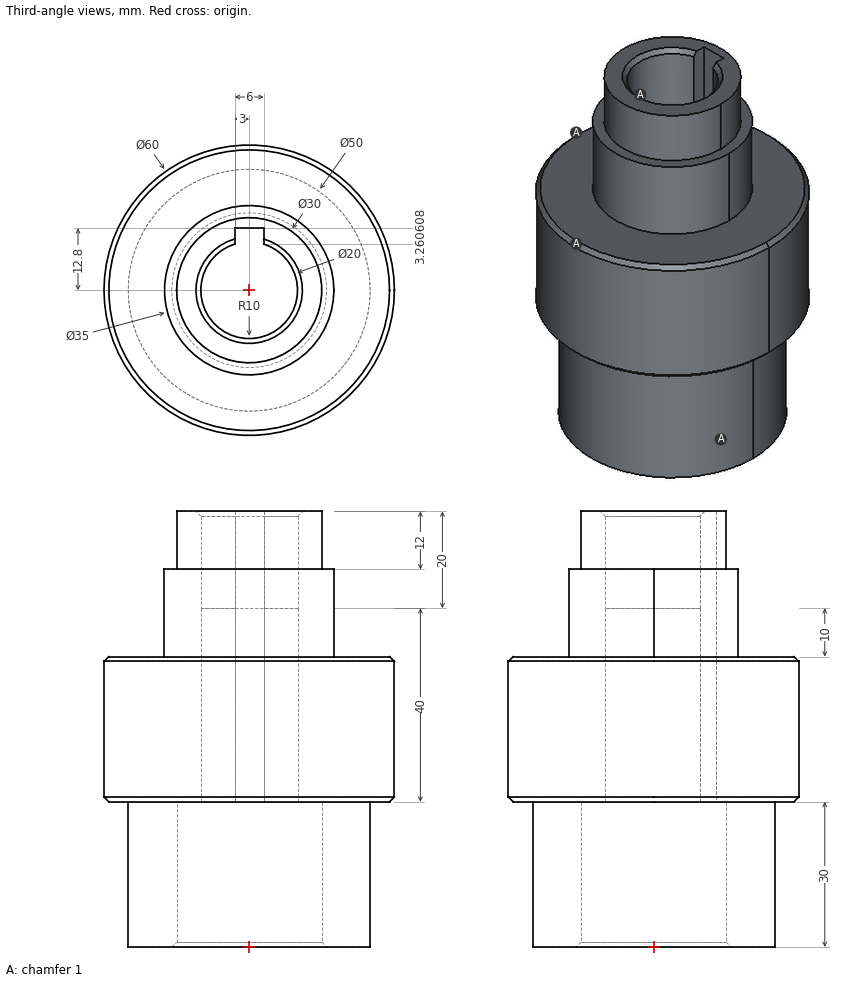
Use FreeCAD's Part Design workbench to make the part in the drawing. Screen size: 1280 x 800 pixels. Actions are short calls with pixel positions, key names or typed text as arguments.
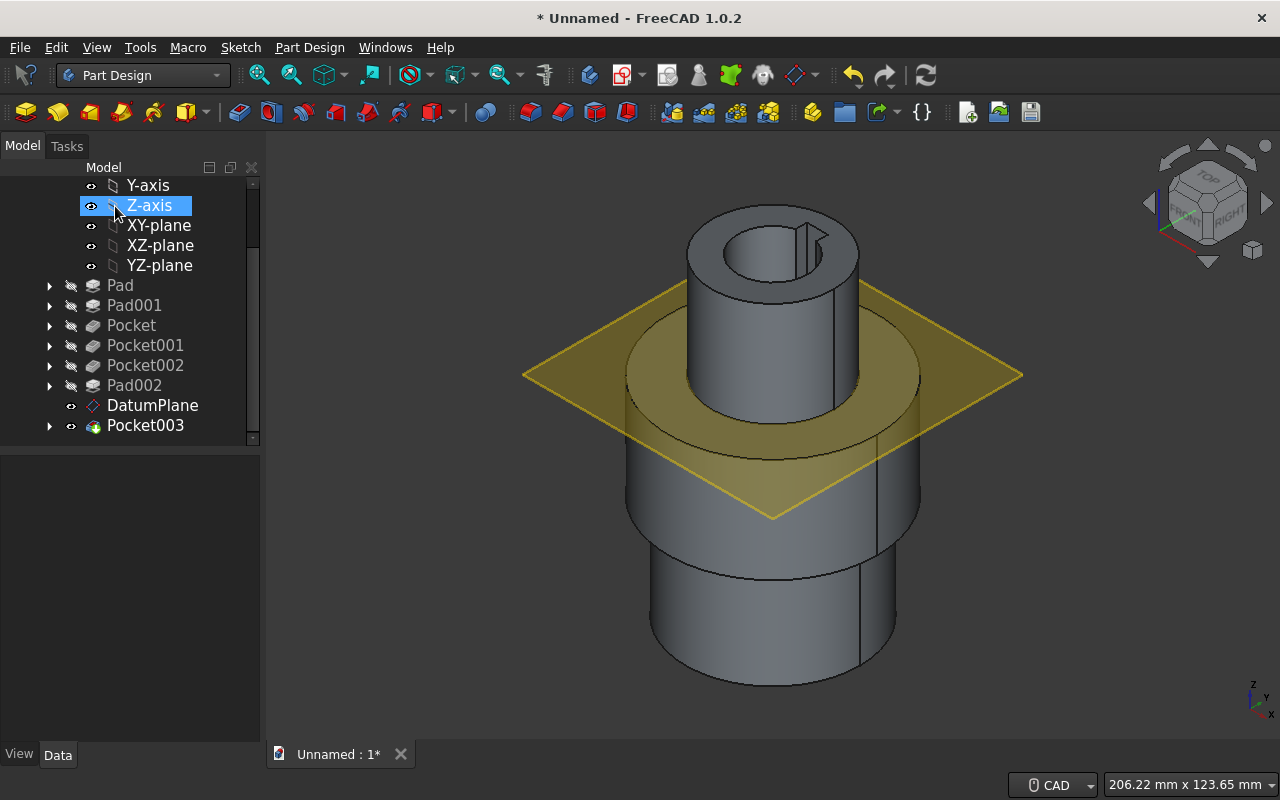
click(116, 406)
key(space)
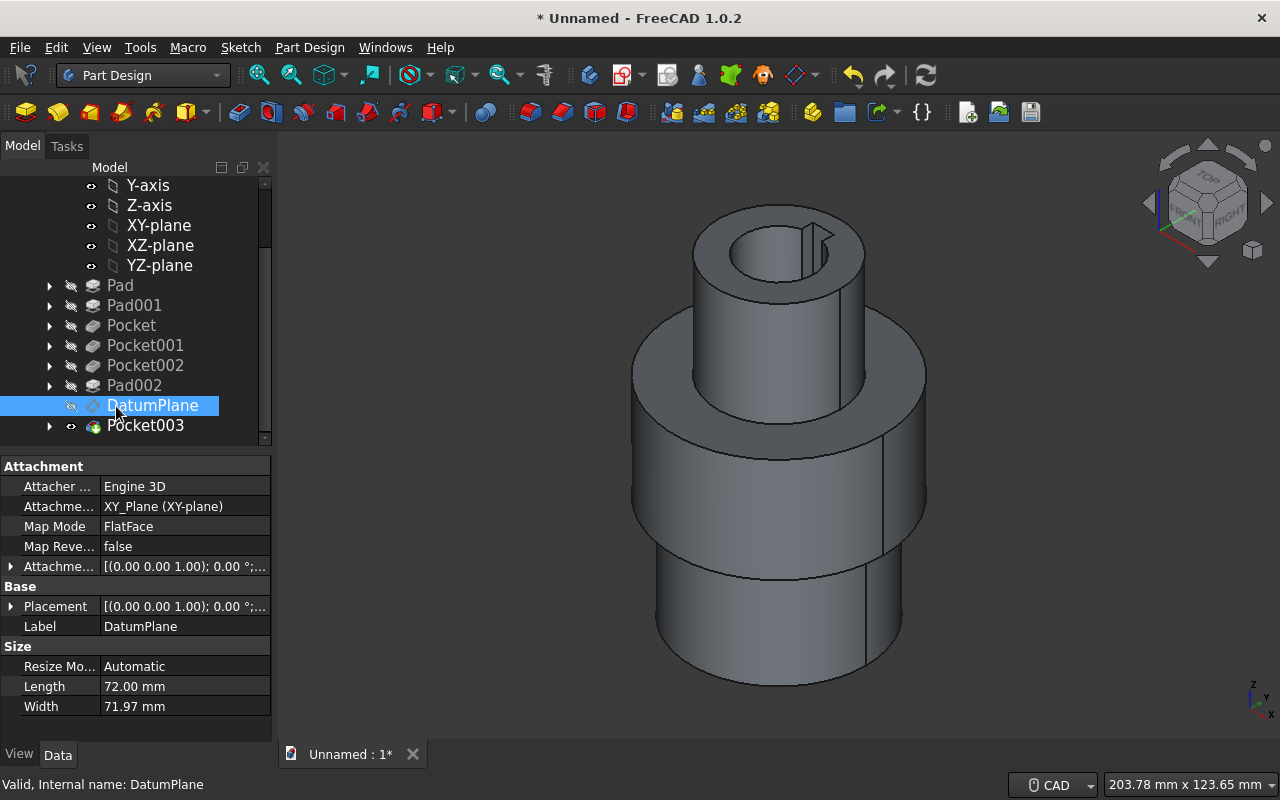
scroll(160, 301, down, 3)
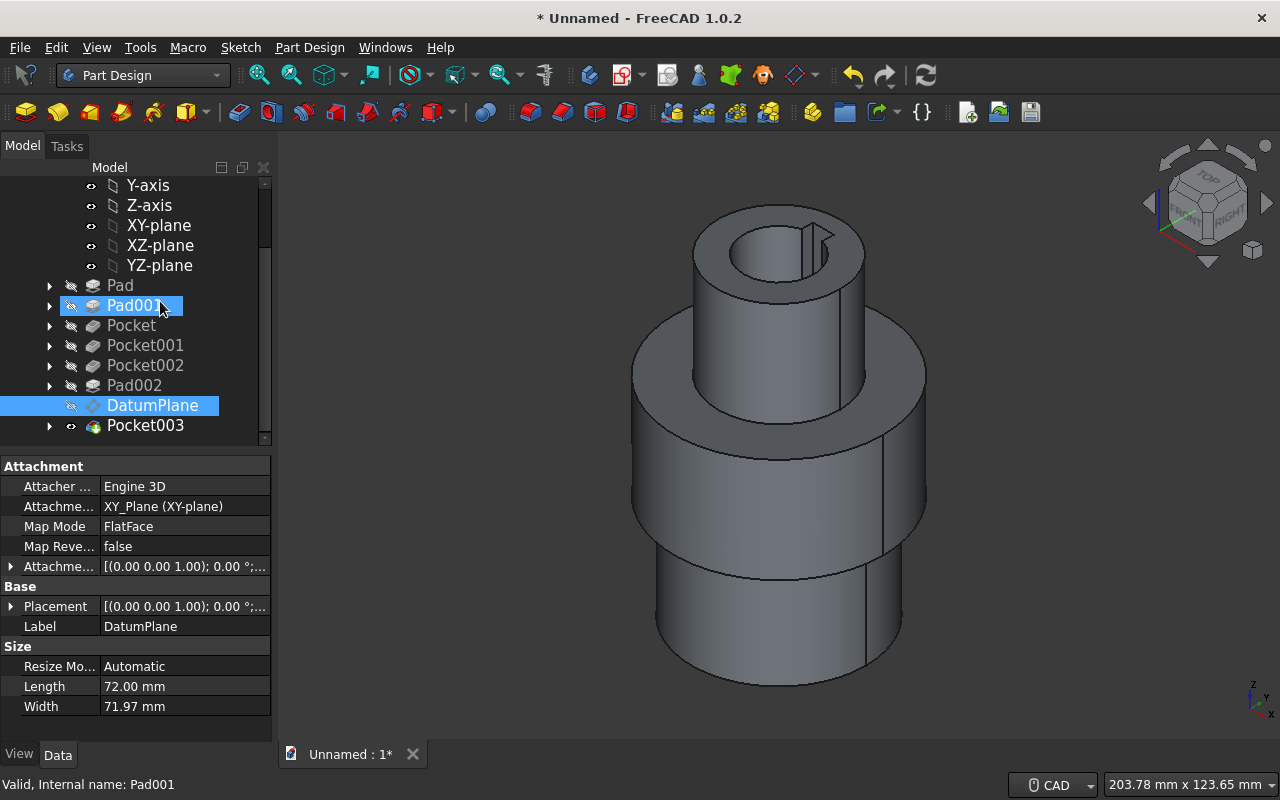
scroll(160, 301, up, 15)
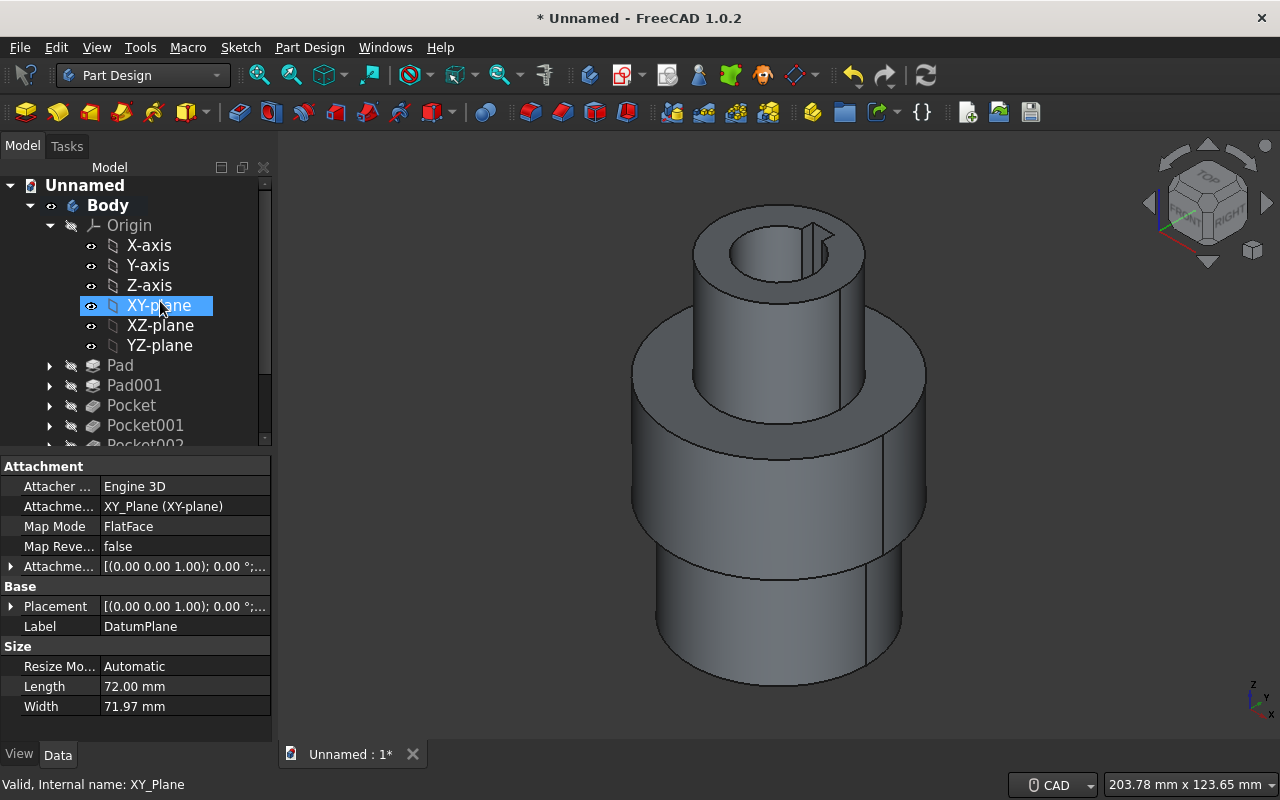
click(136, 306)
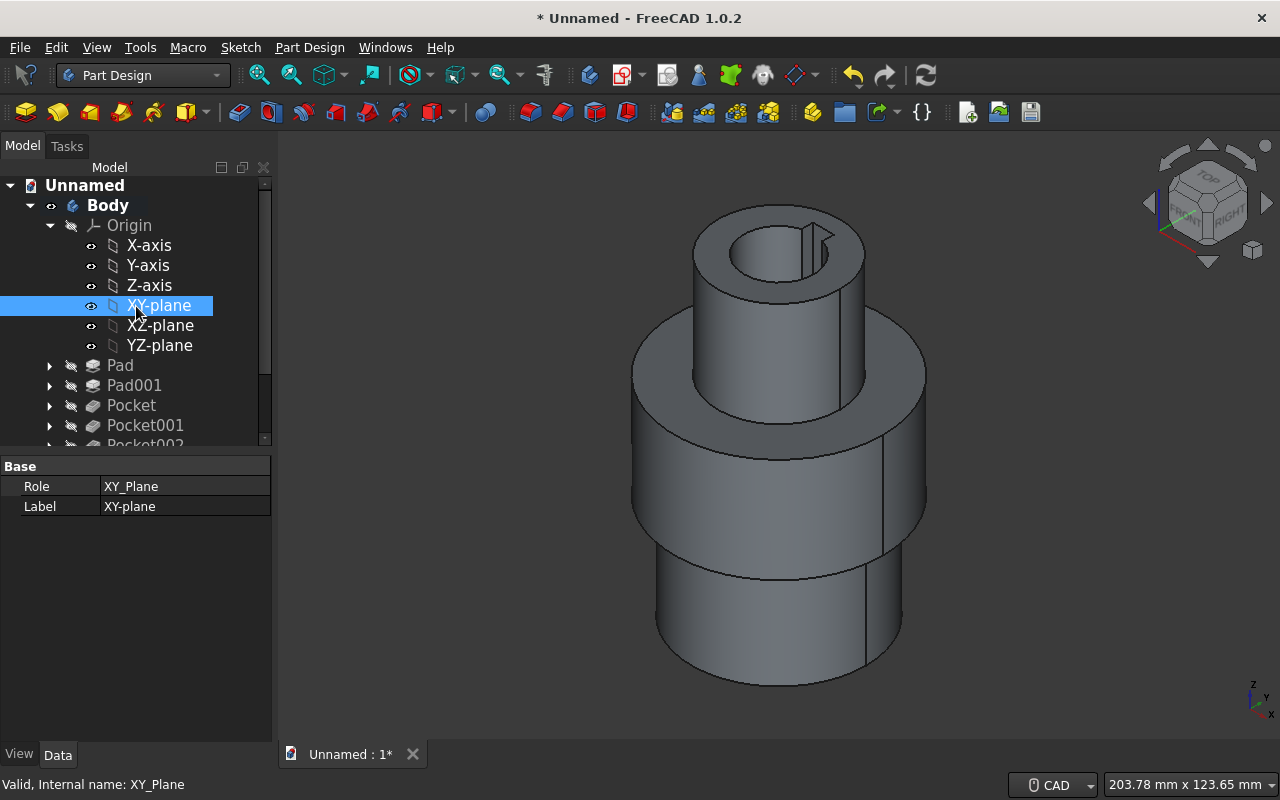
click(796, 76)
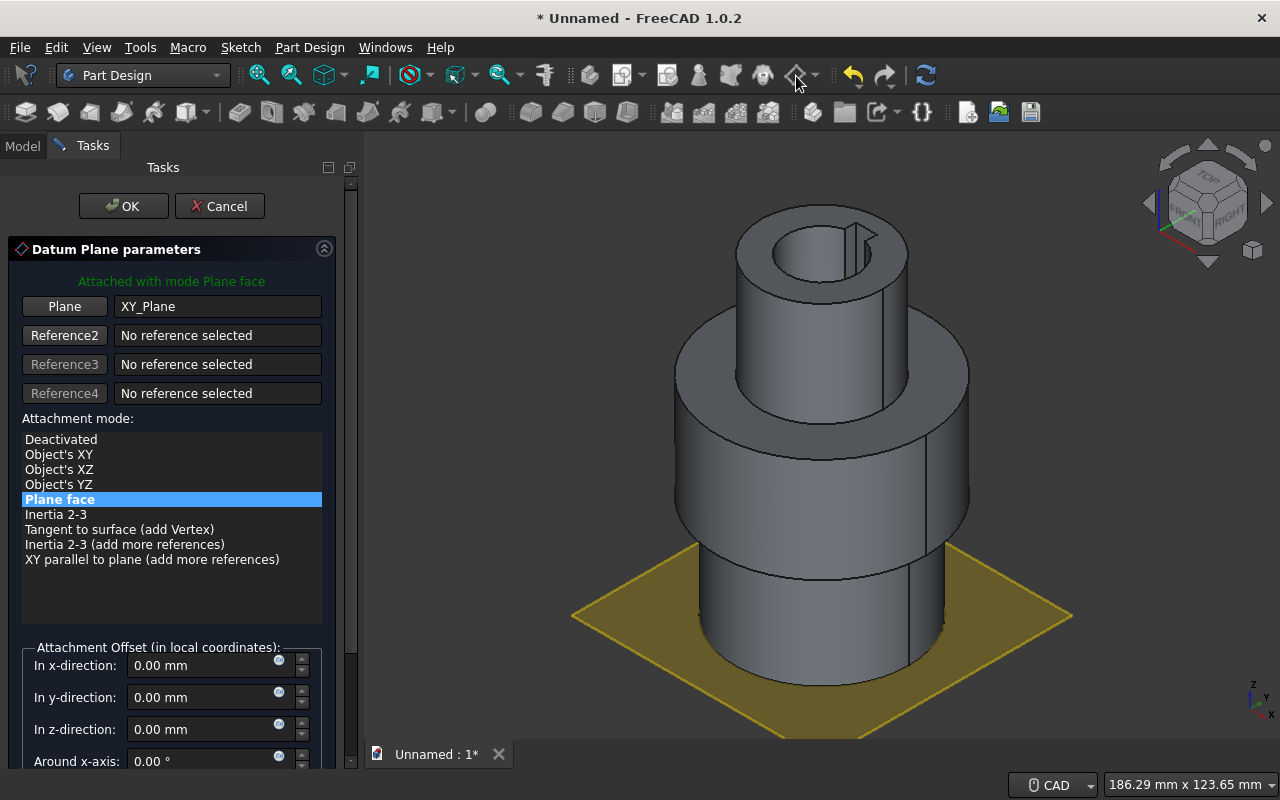
triple_click(210, 729)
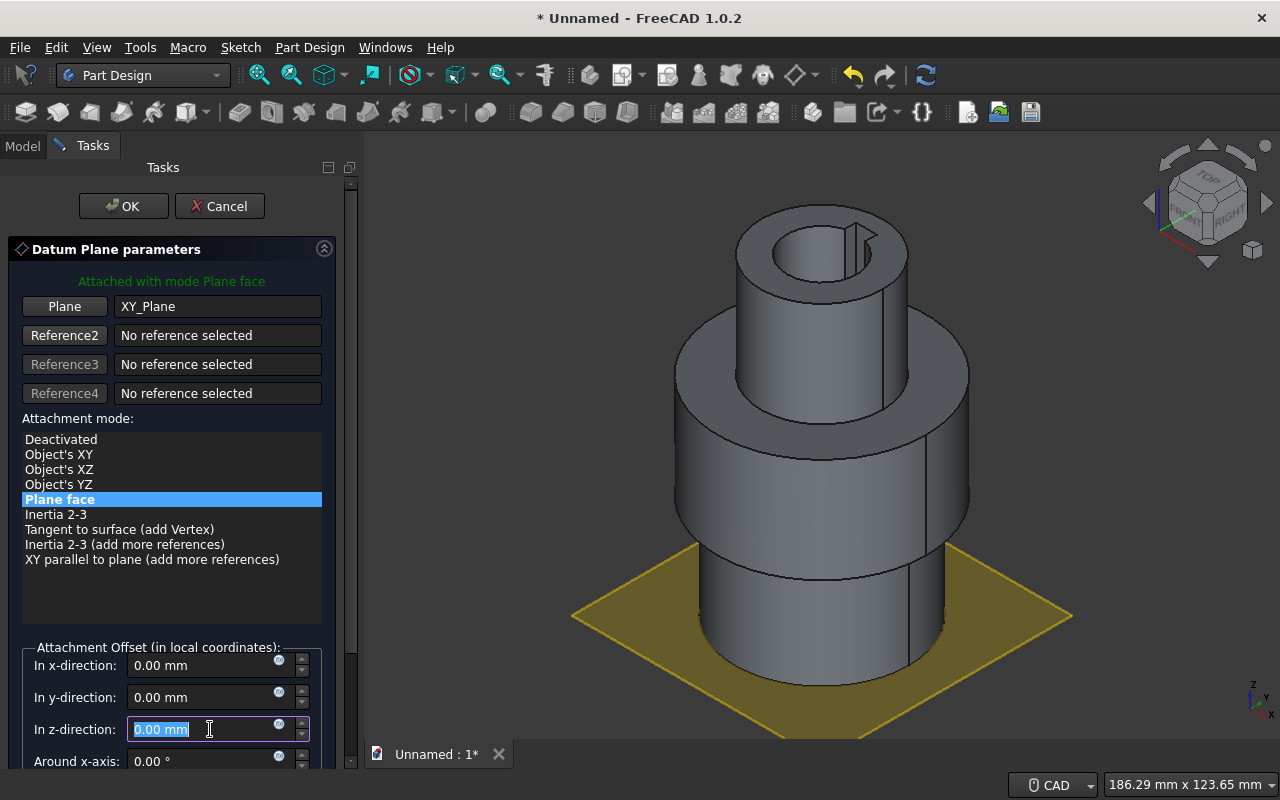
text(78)
key(Tab)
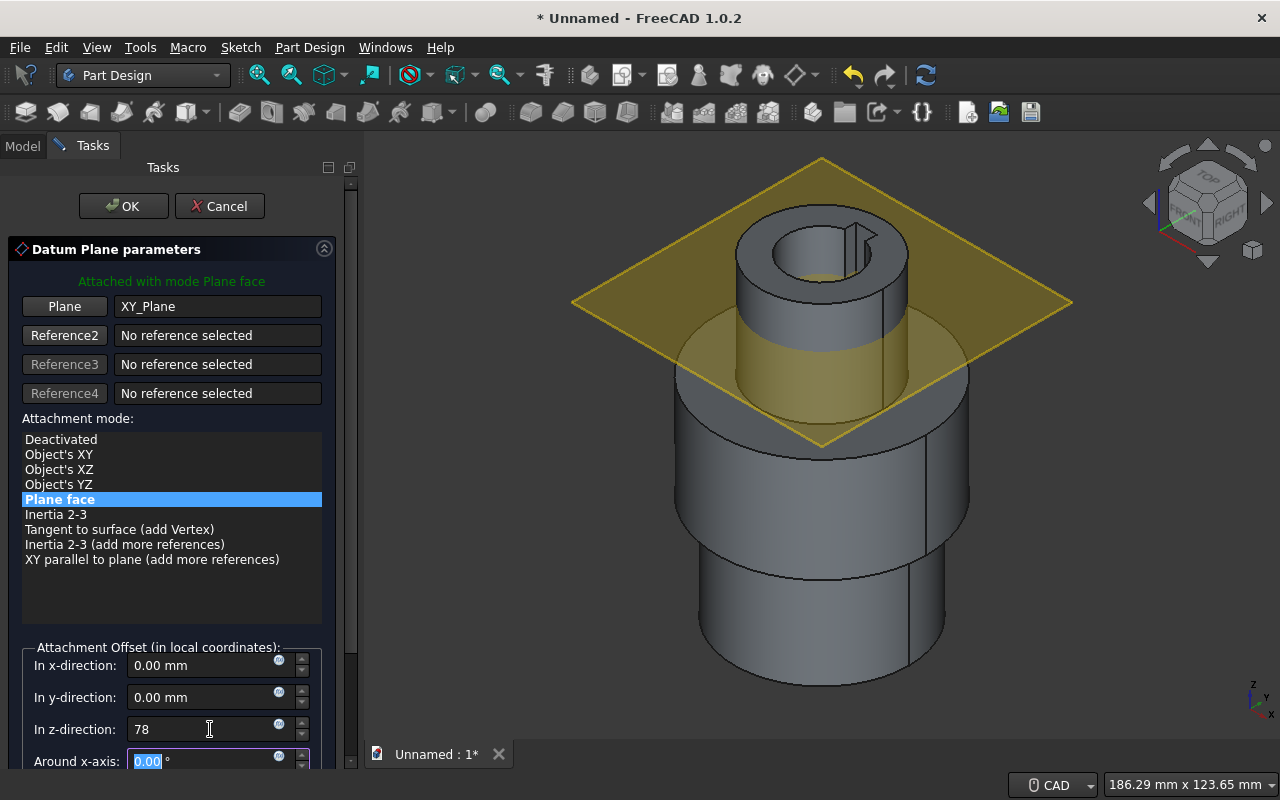
click(124, 206)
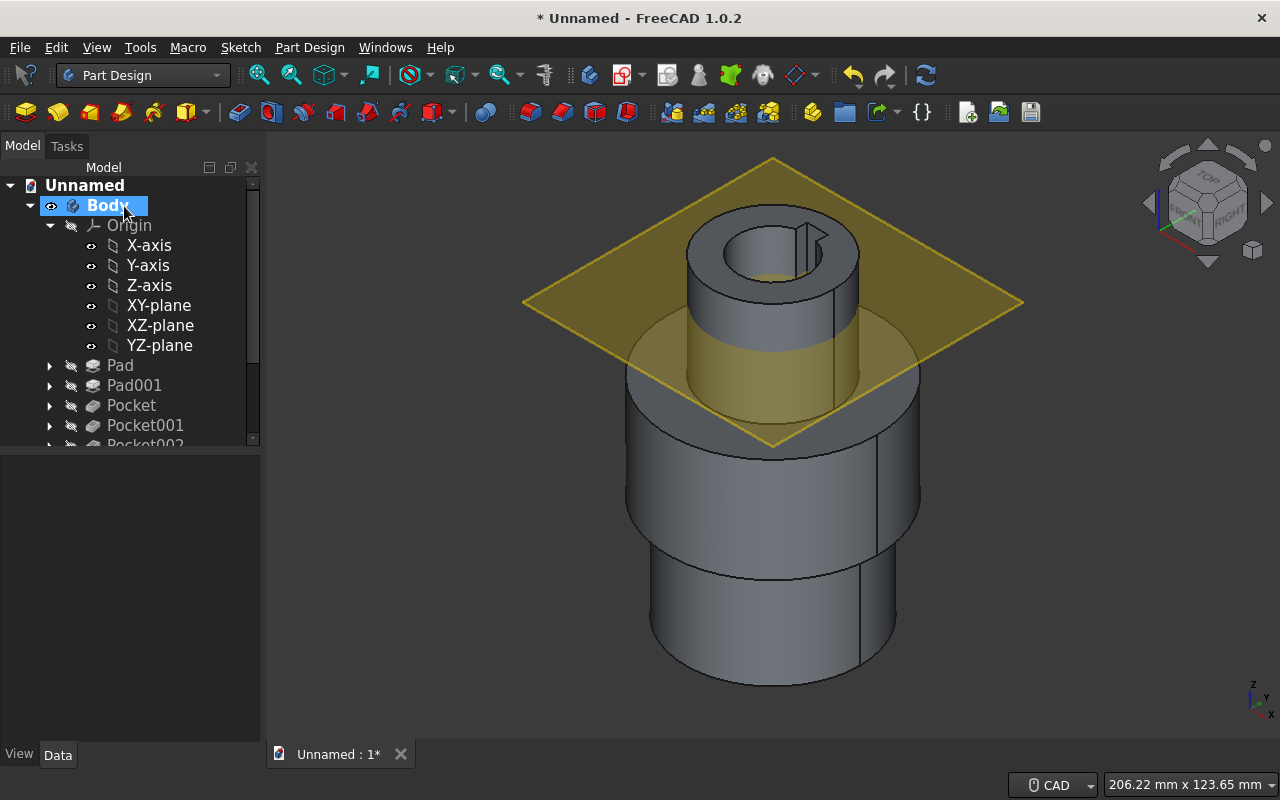
scroll(100, 321, down, 3)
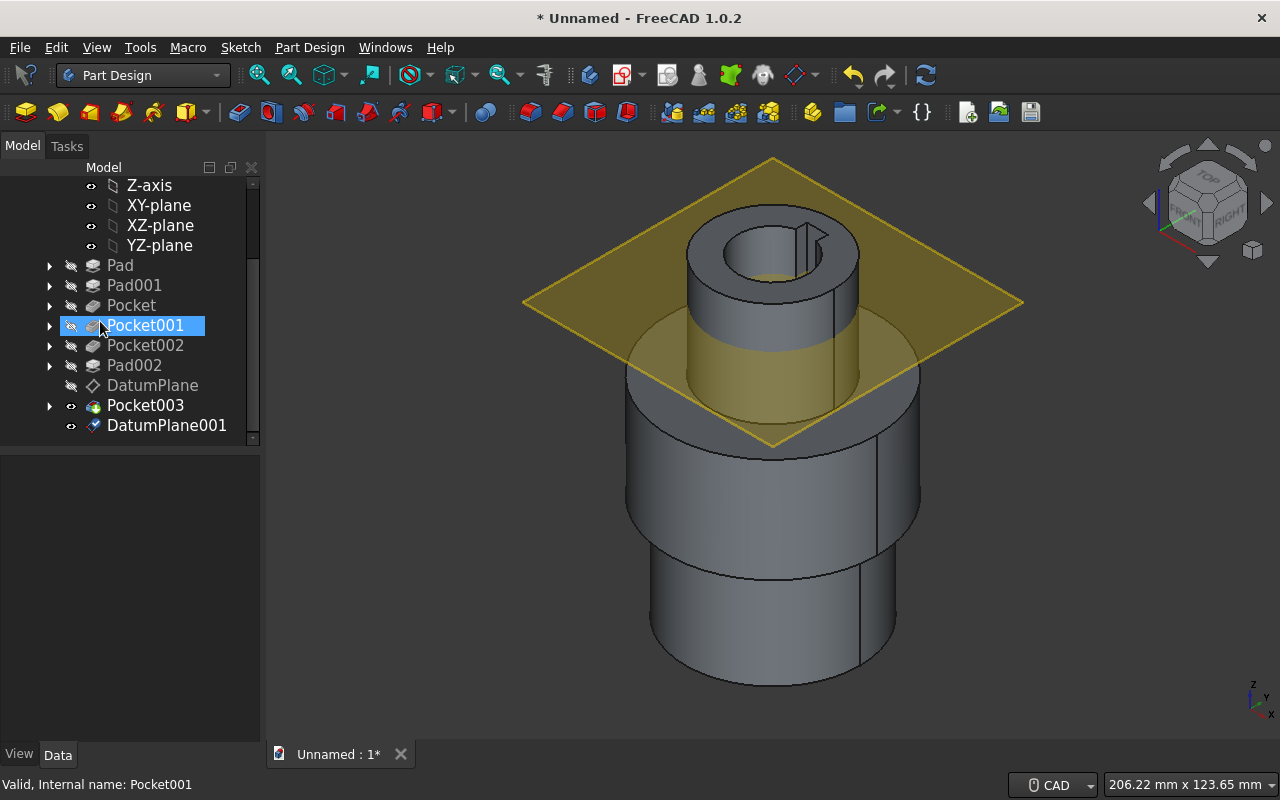
click(116, 426)